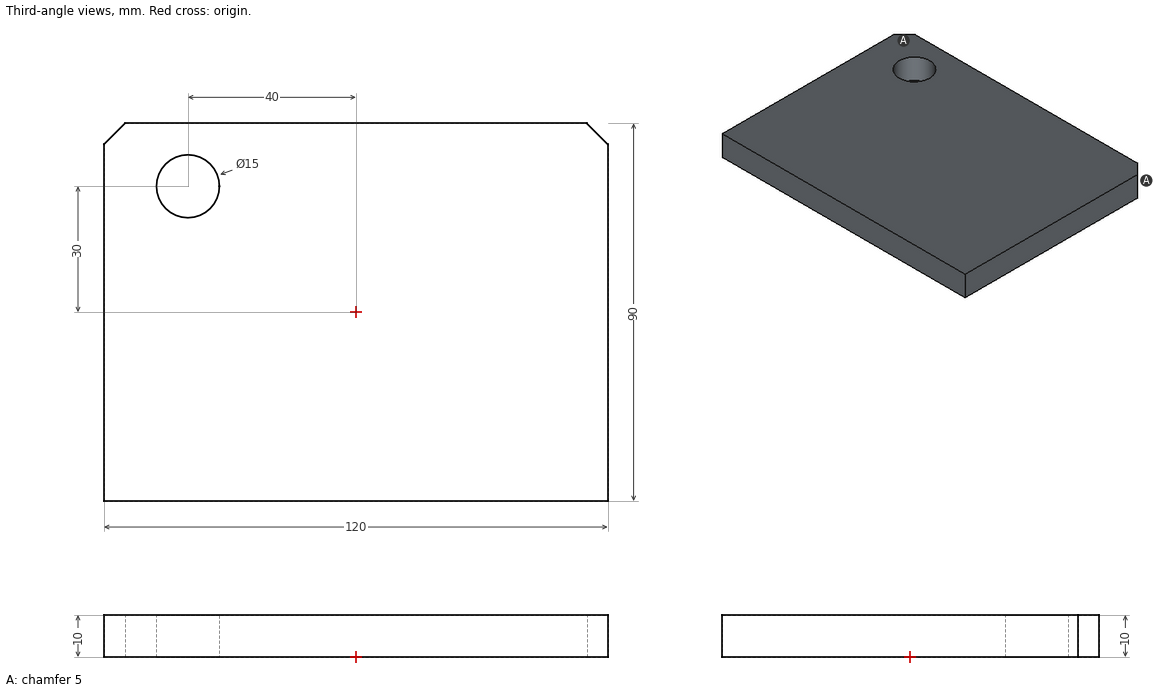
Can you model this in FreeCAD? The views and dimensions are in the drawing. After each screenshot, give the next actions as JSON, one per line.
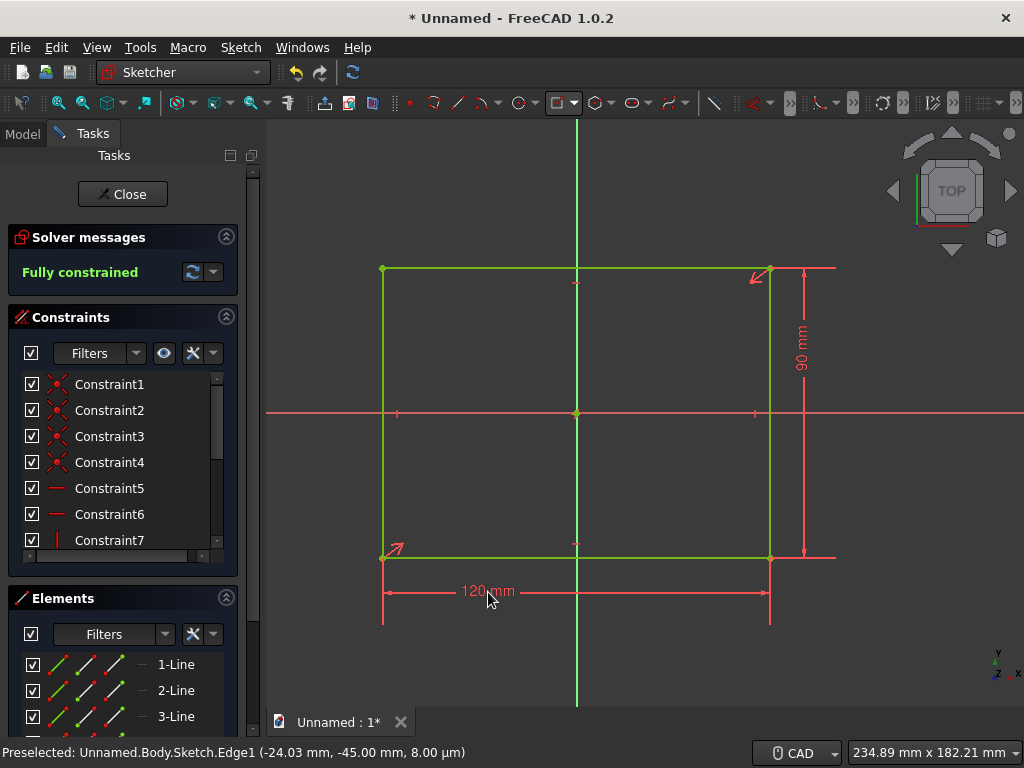
{"action": "left_click", "coordinate": [123, 194]}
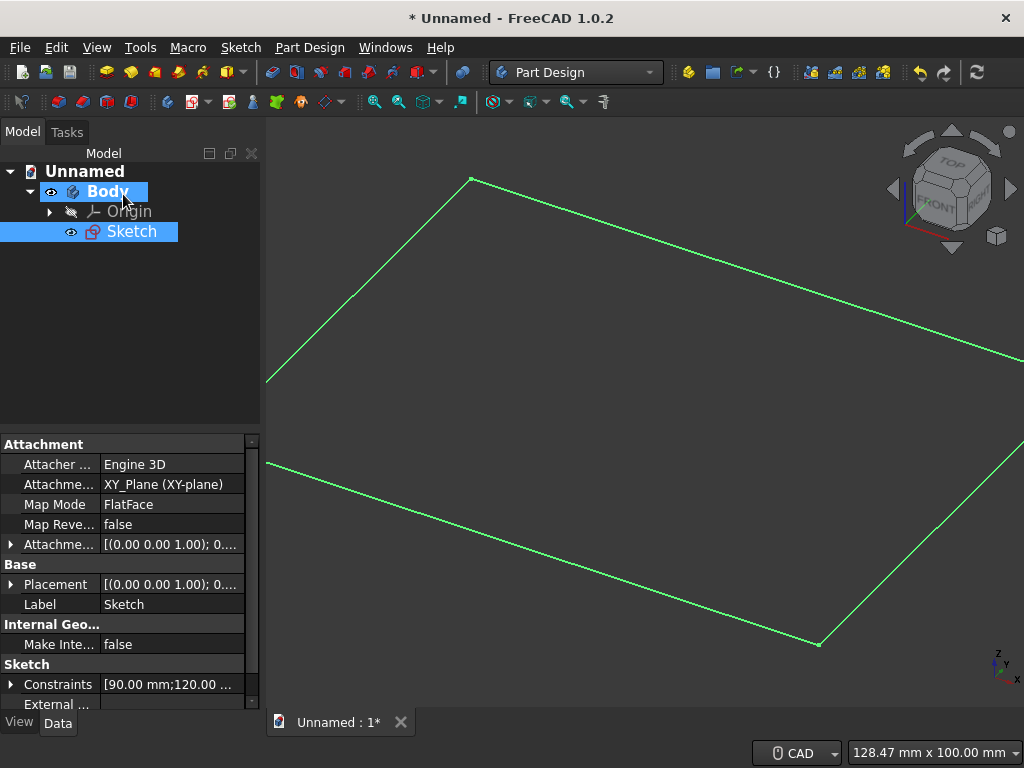
{"action": "left_click", "coordinate": [108, 72]}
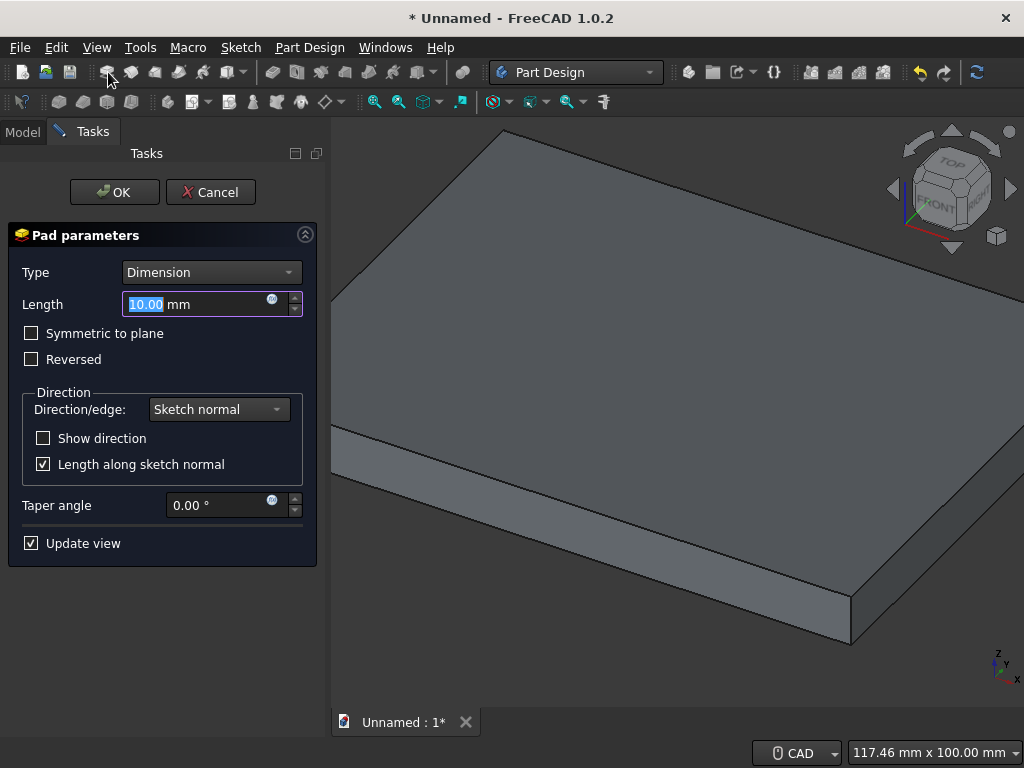
{"action": "type", "text": "10"}
{"action": "key", "text": "Tab"}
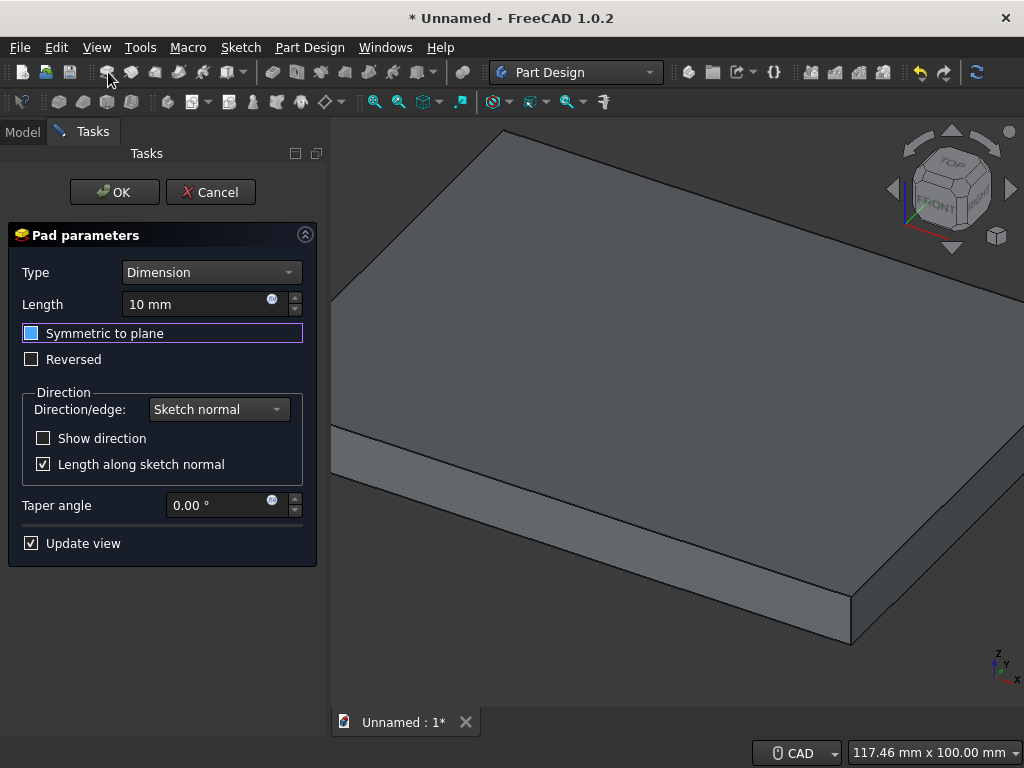
{"action": "left_click", "coordinate": [115, 192]}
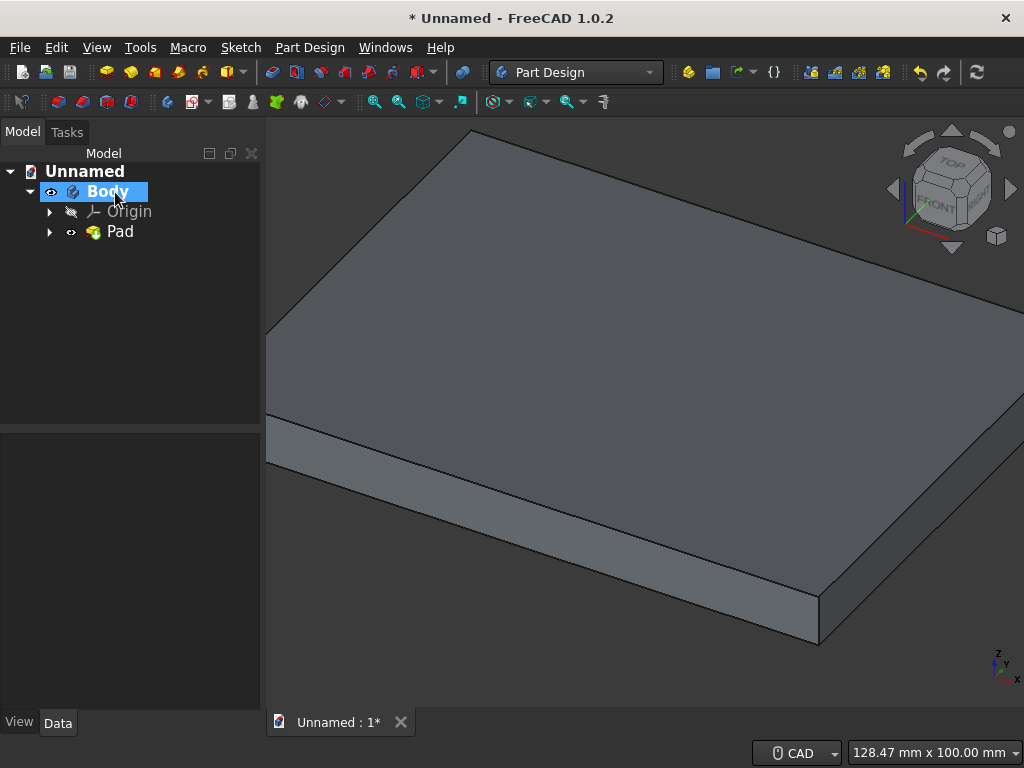
{"action": "left_click", "coordinate": [376, 102]}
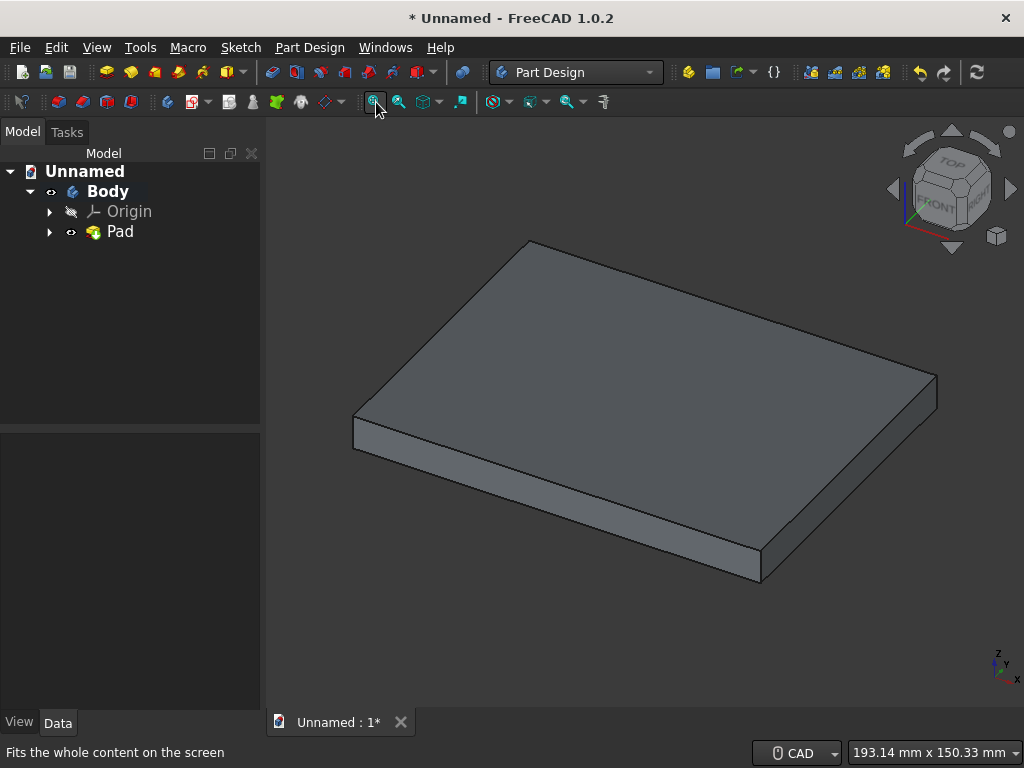
{"action": "left_click", "coordinate": [645, 395]}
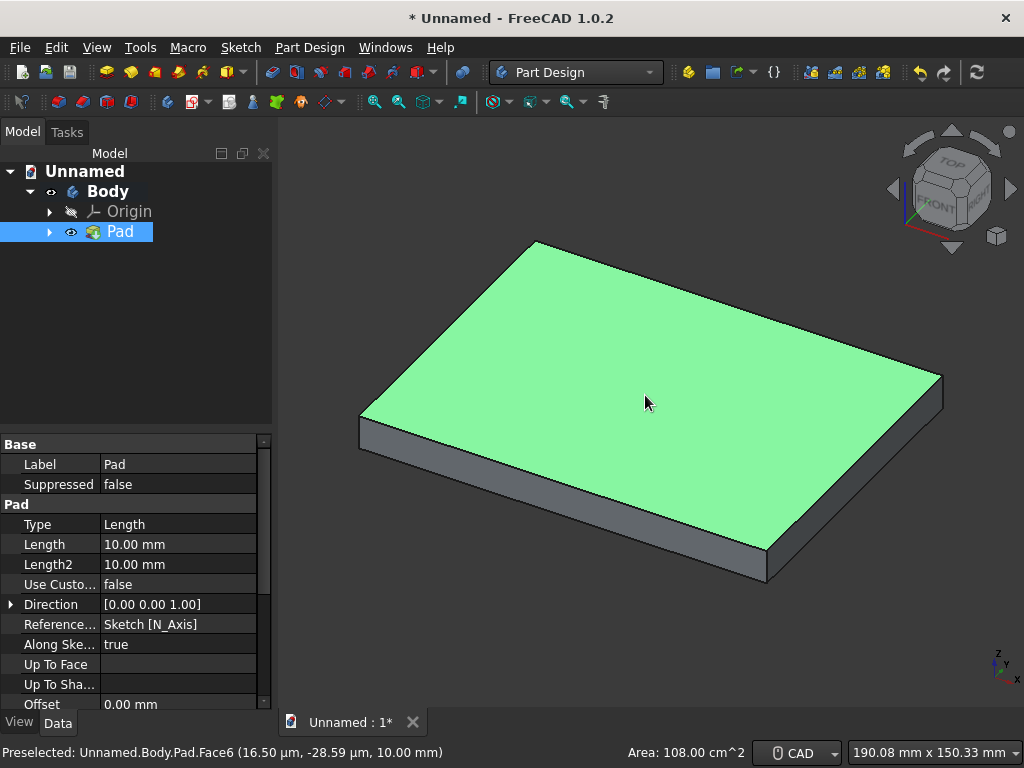
{"action": "left_click", "coordinate": [192, 102]}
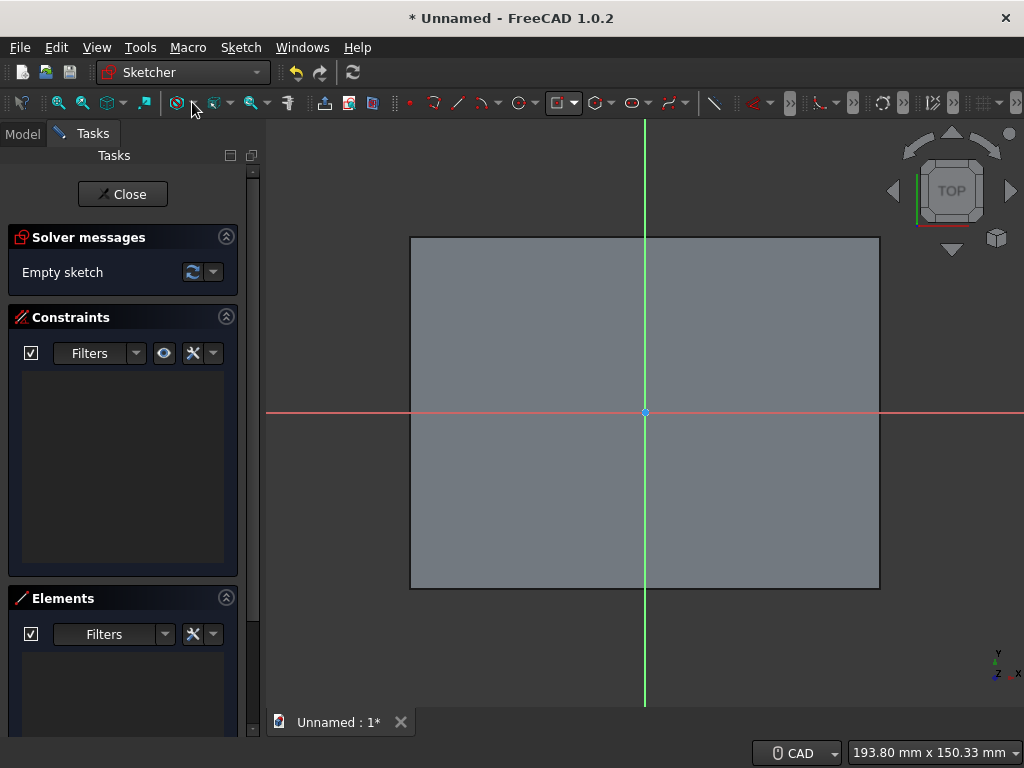
{"action": "scroll", "coordinate": [471, 272], "scroll_direction": "up", "scroll_amount": 9}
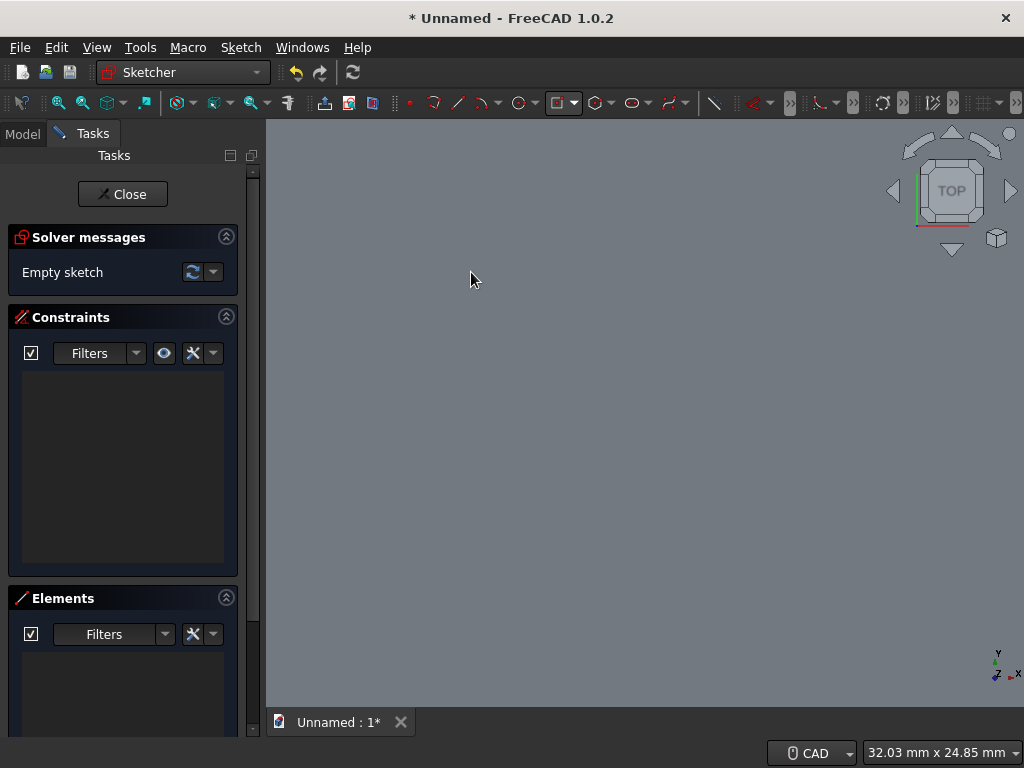
{"action": "left_click", "coordinate": [520, 104]}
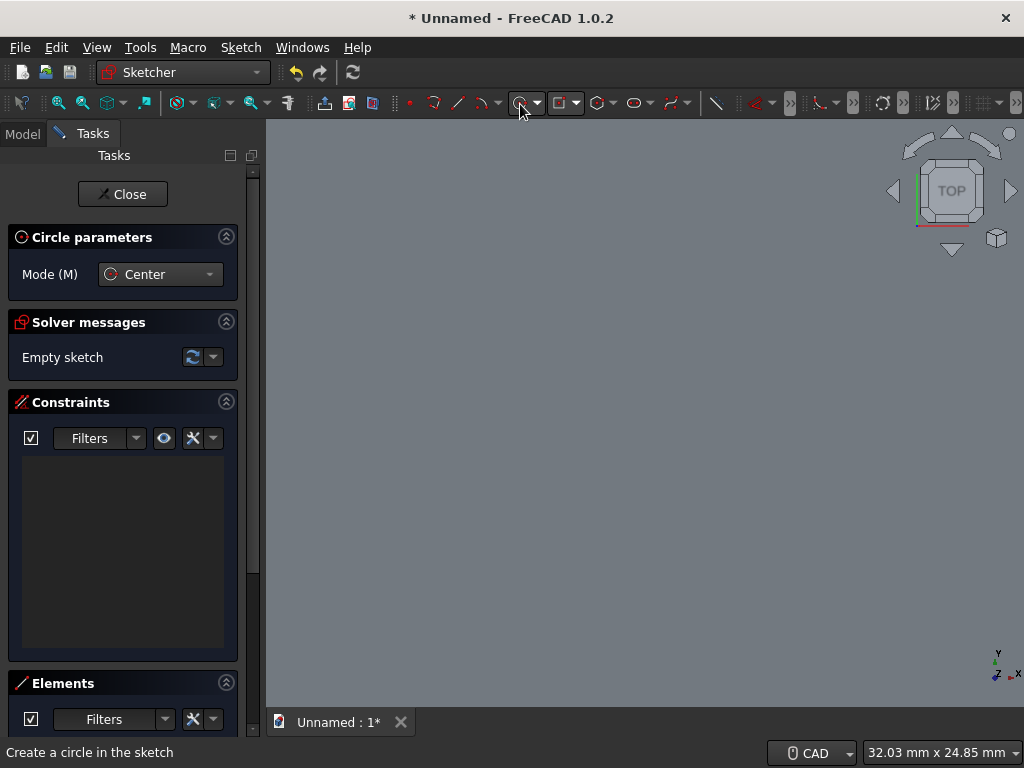
{"action": "left_click", "coordinate": [576, 414]}
{"action": "left_click", "coordinate": [701, 288]}
{"action": "key", "text": "Escape"}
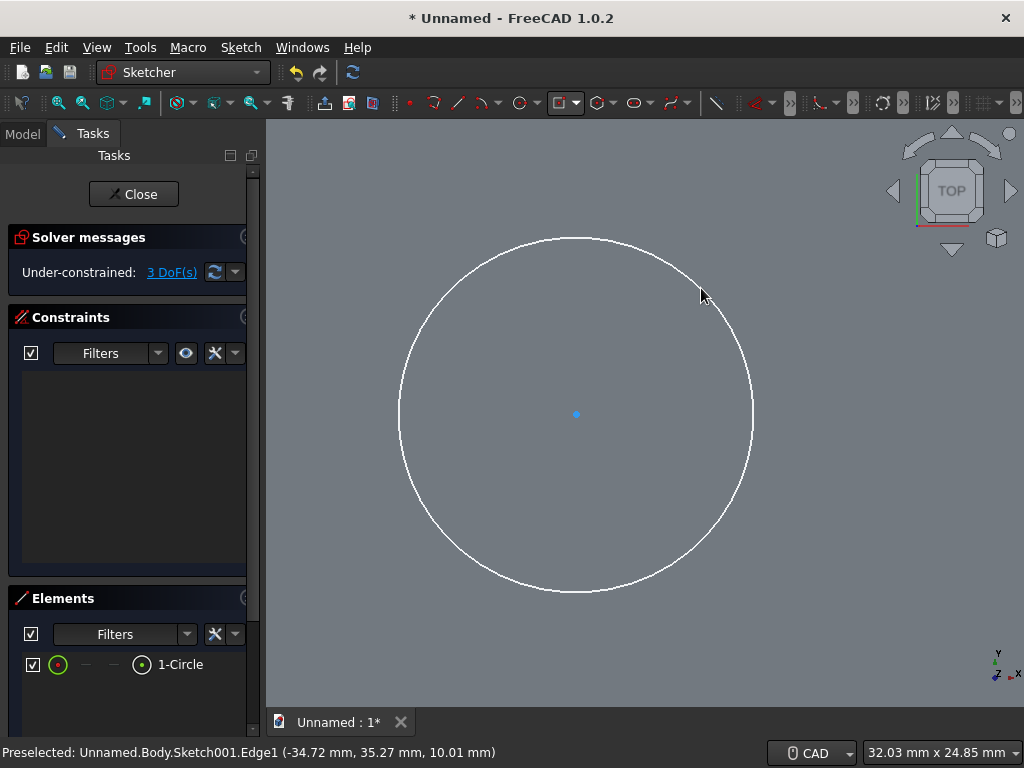
{"action": "left_click", "coordinate": [756, 104]}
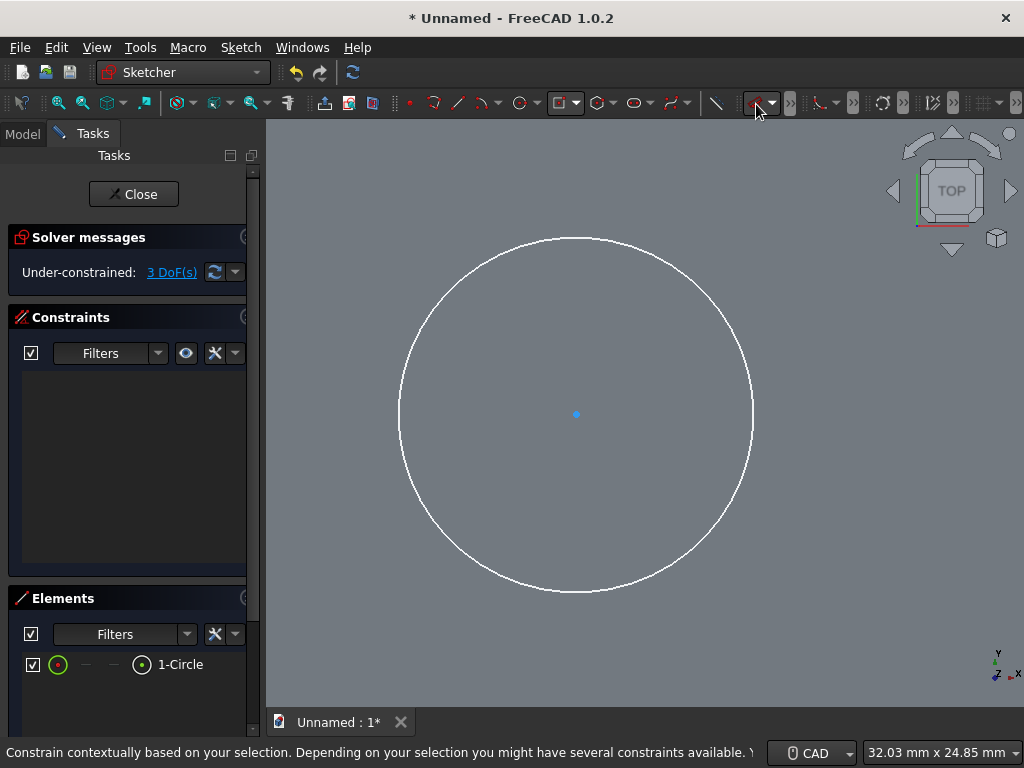
{"action": "left_click", "coordinate": [701, 289]}
{"action": "left_click", "coordinate": [724, 266]}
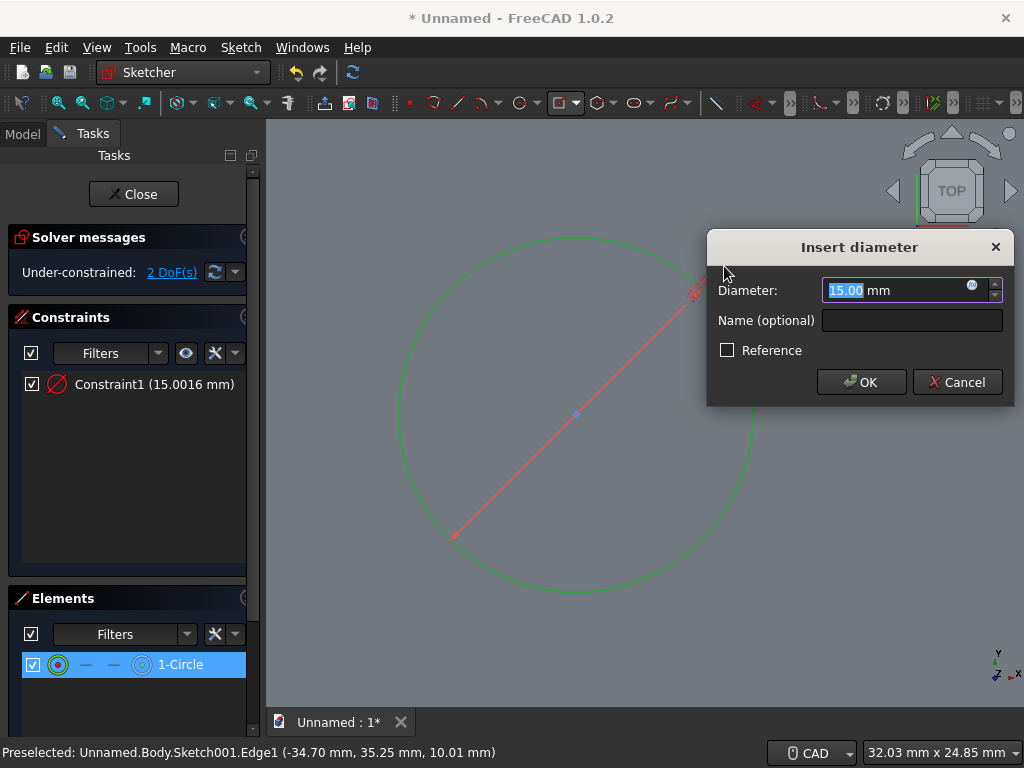
{"action": "type", "text": "15"}
{"action": "key", "text": "Return"}